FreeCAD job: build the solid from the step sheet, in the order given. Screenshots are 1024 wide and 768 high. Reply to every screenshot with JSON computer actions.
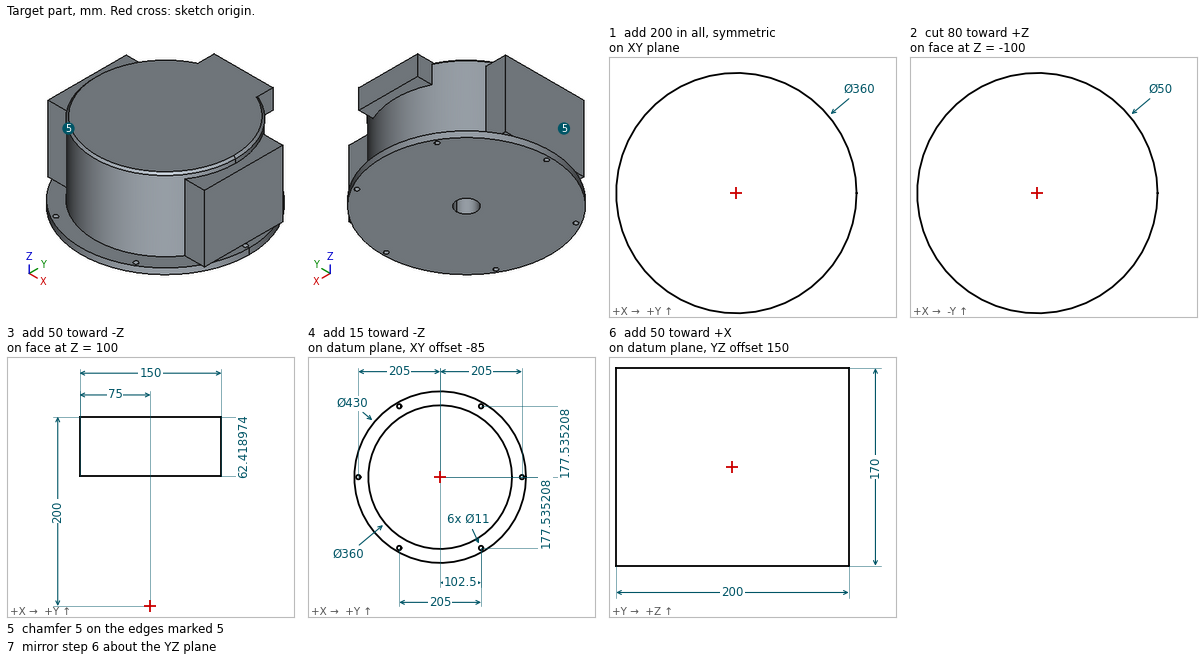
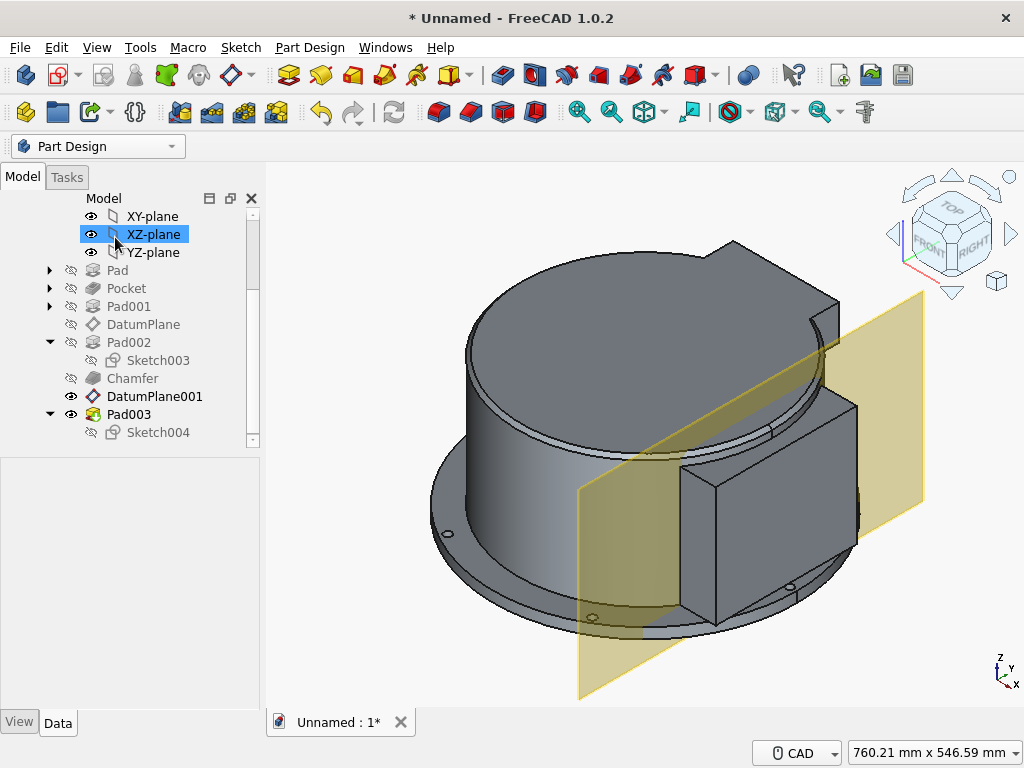
{"action": "left_click", "coordinate": [116, 396]}
{"action": "key", "text": "space"}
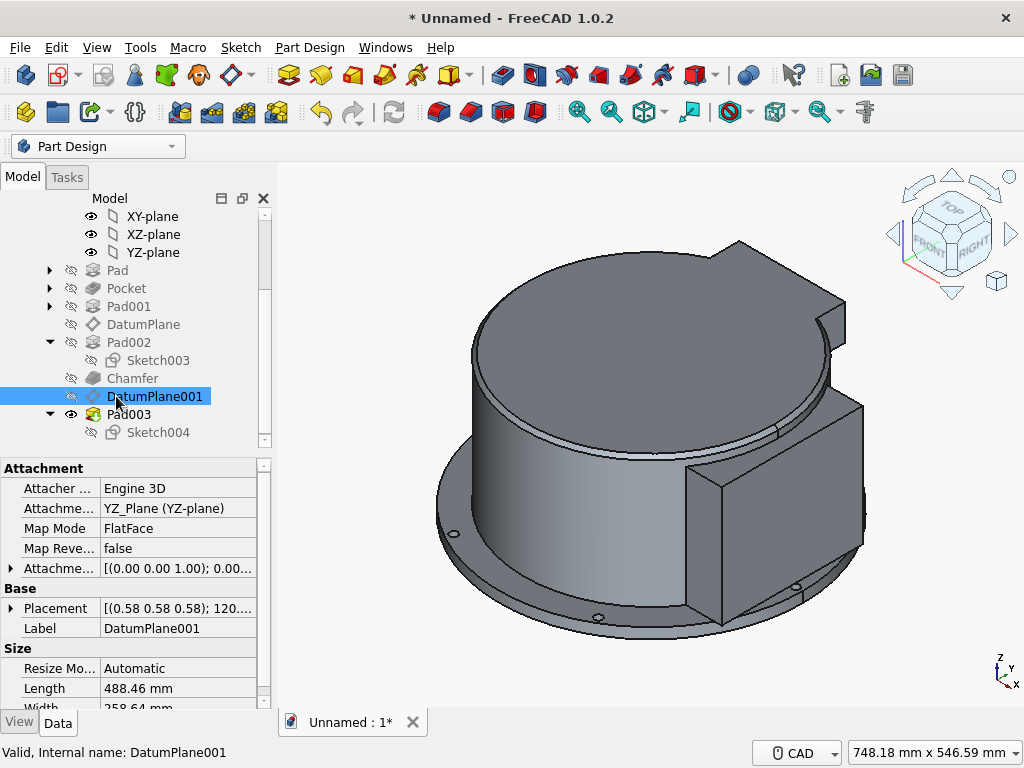
{"action": "left_click", "coordinate": [116, 414]}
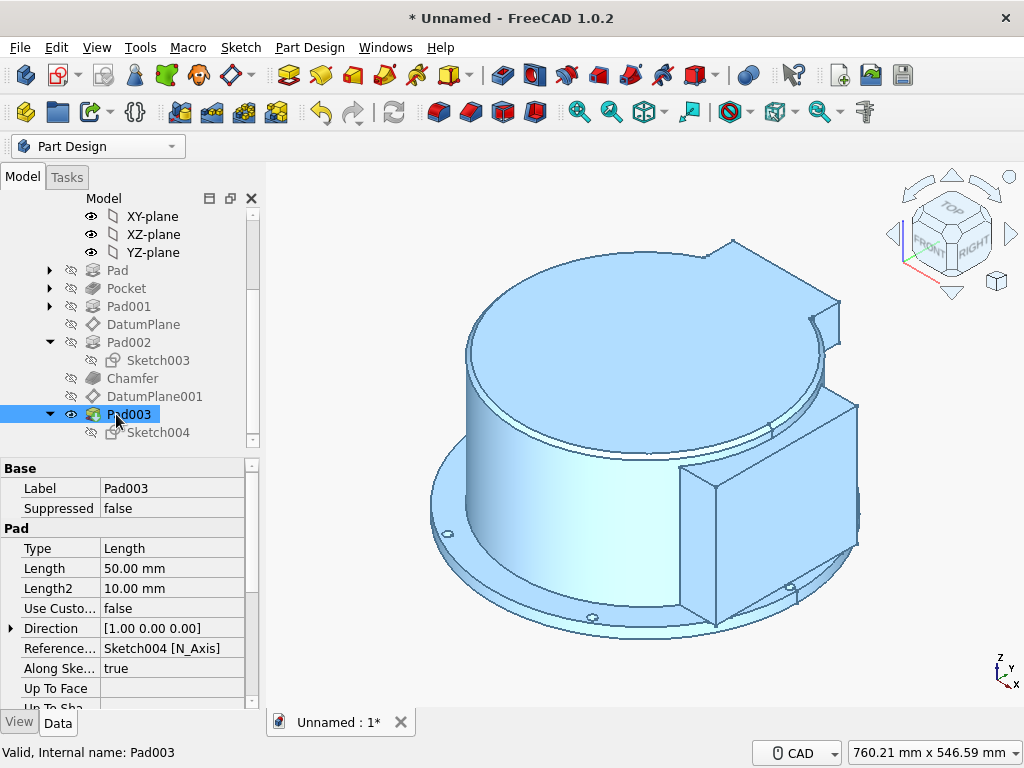
{"action": "left_click", "coordinate": [180, 112]}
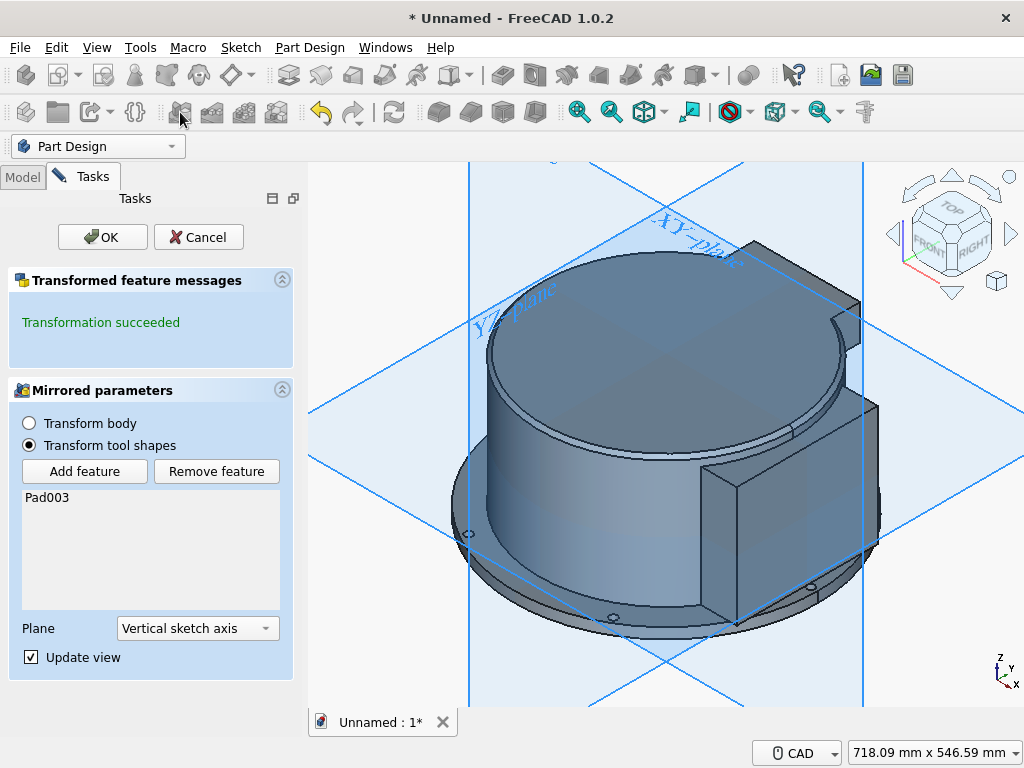
{"action": "left_click", "coordinate": [198, 628]}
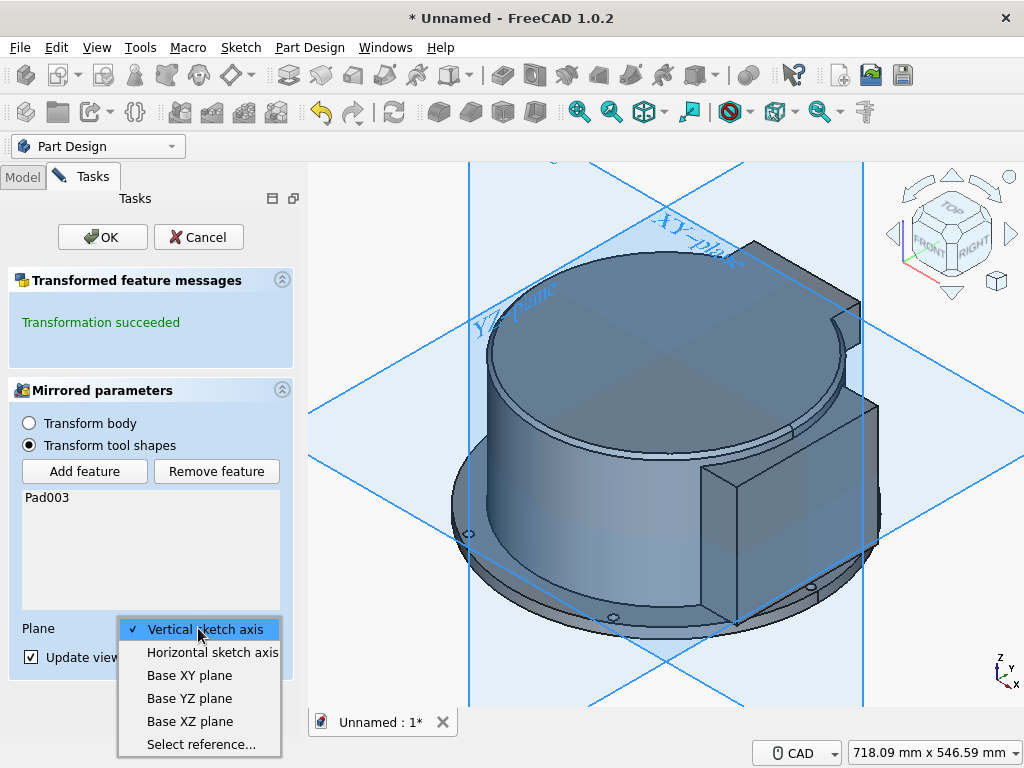
{"action": "left_click", "coordinate": [198, 698]}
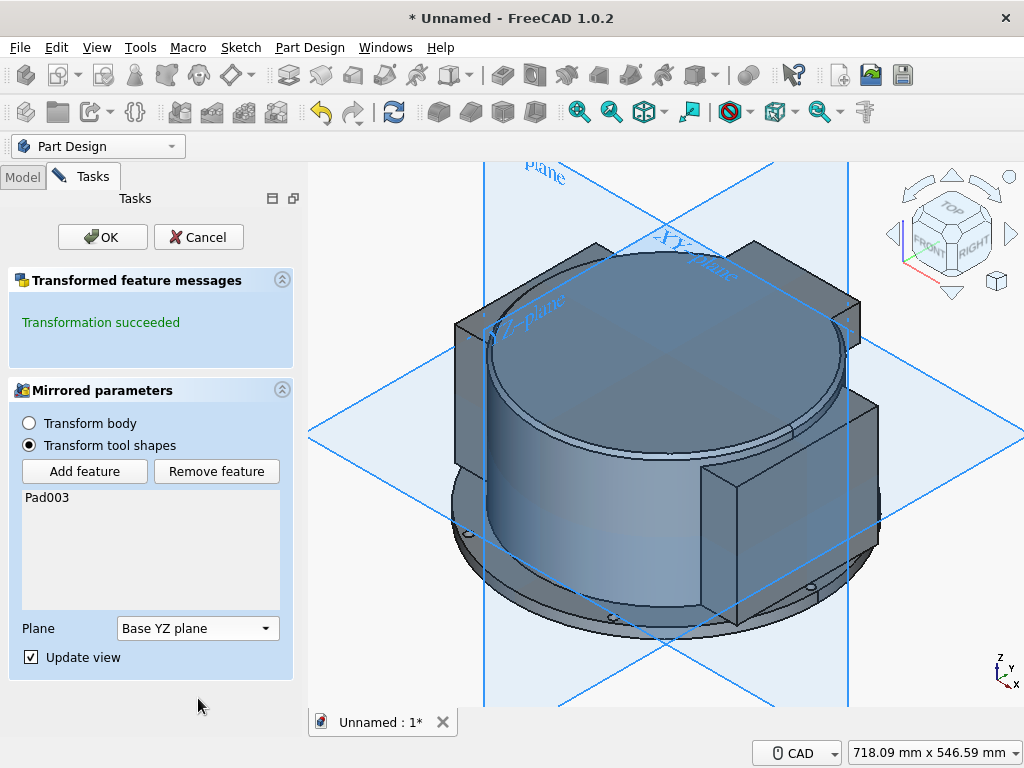
{"action": "left_click", "coordinate": [103, 237]}